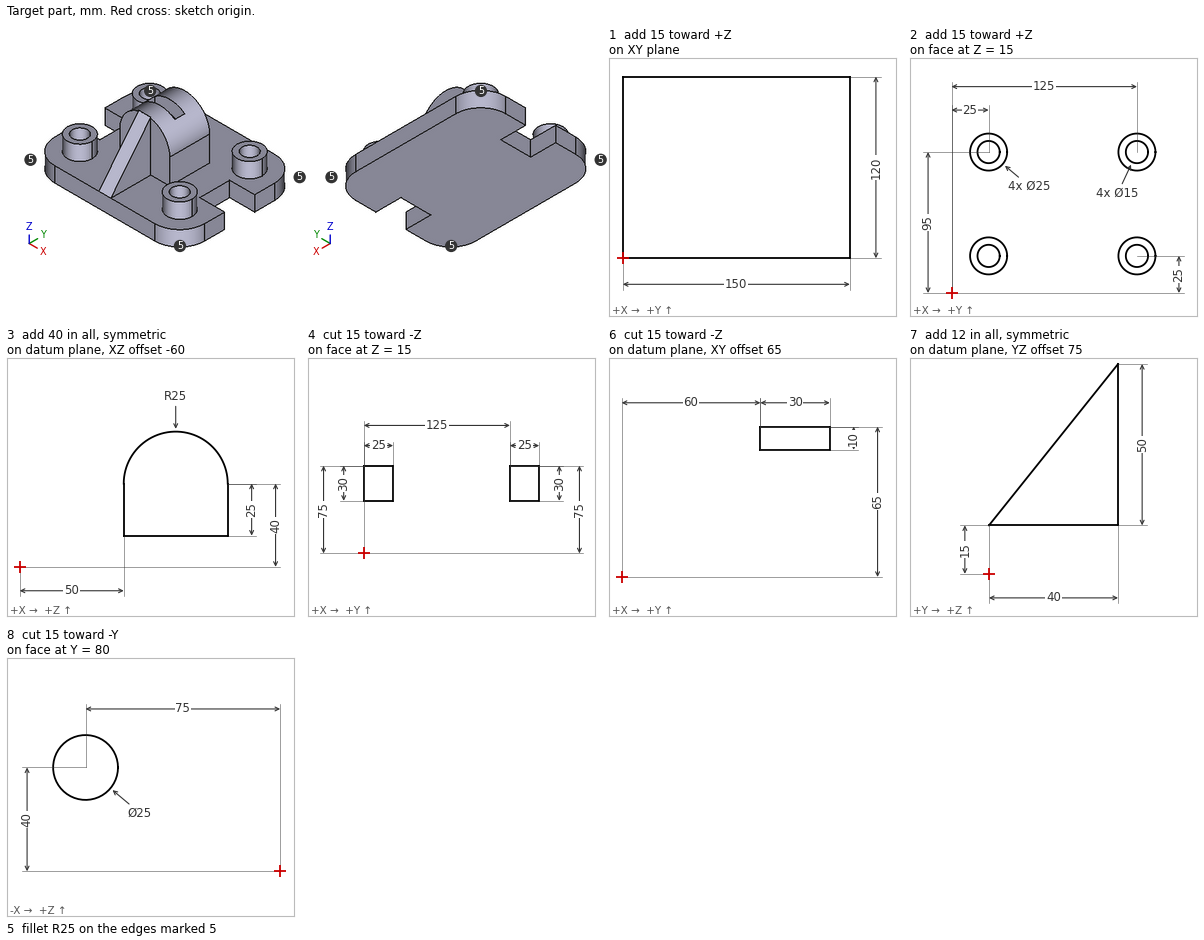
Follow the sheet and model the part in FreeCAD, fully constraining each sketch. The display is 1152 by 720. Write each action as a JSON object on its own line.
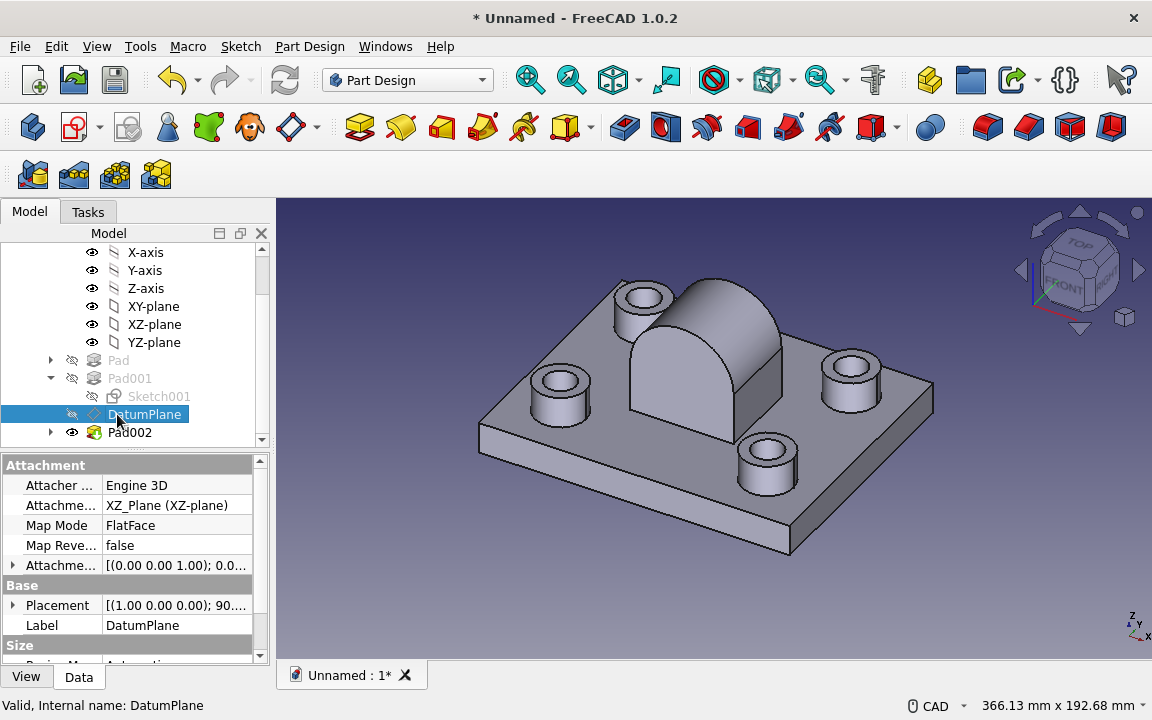
{"action": "left_click", "coordinate": [531, 80]}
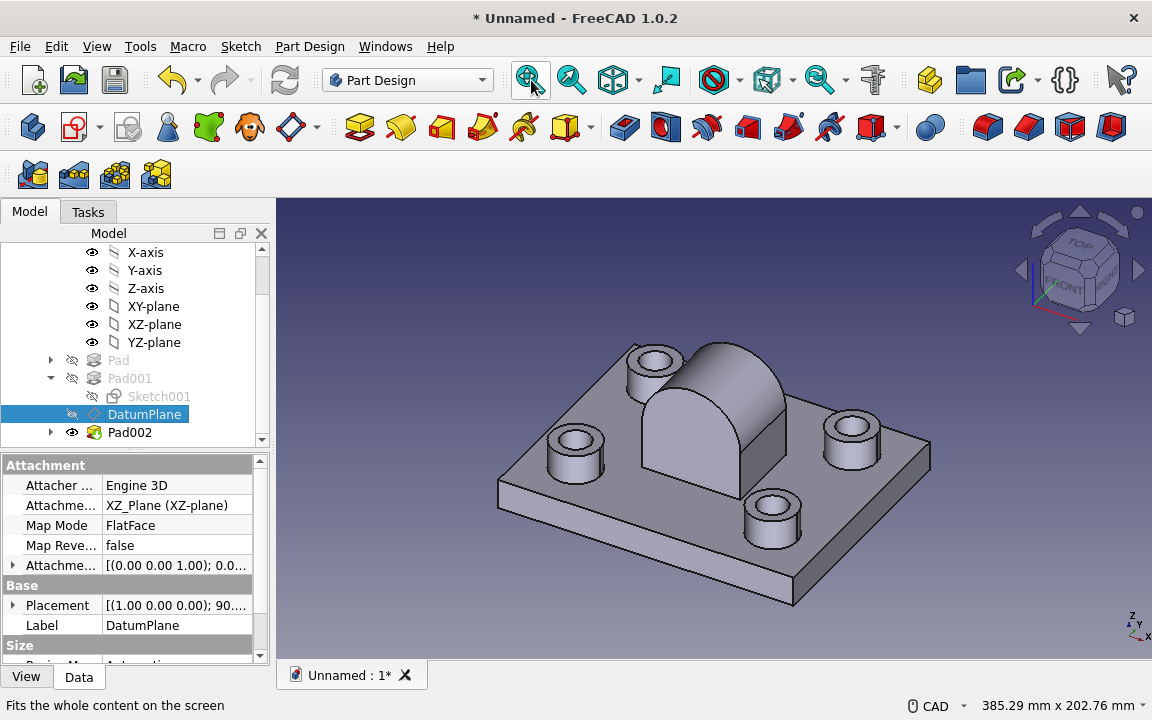
{"action": "left_click", "coordinate": [630, 432]}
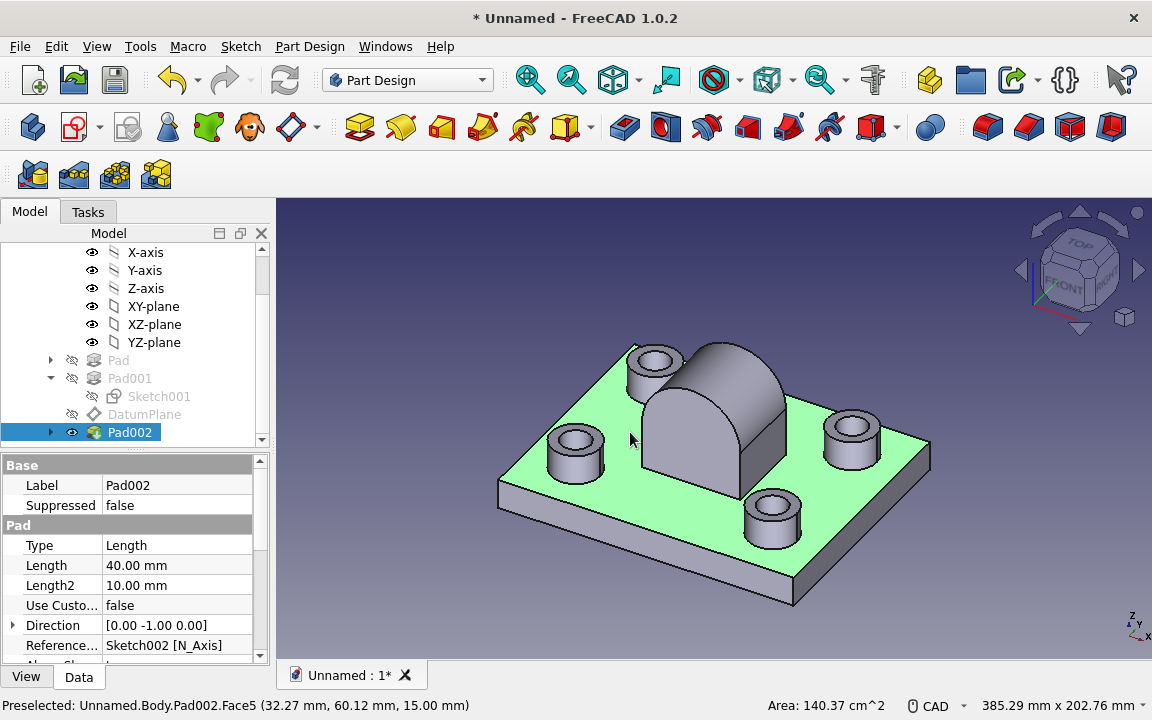
{"action": "left_click", "coordinate": [74, 128]}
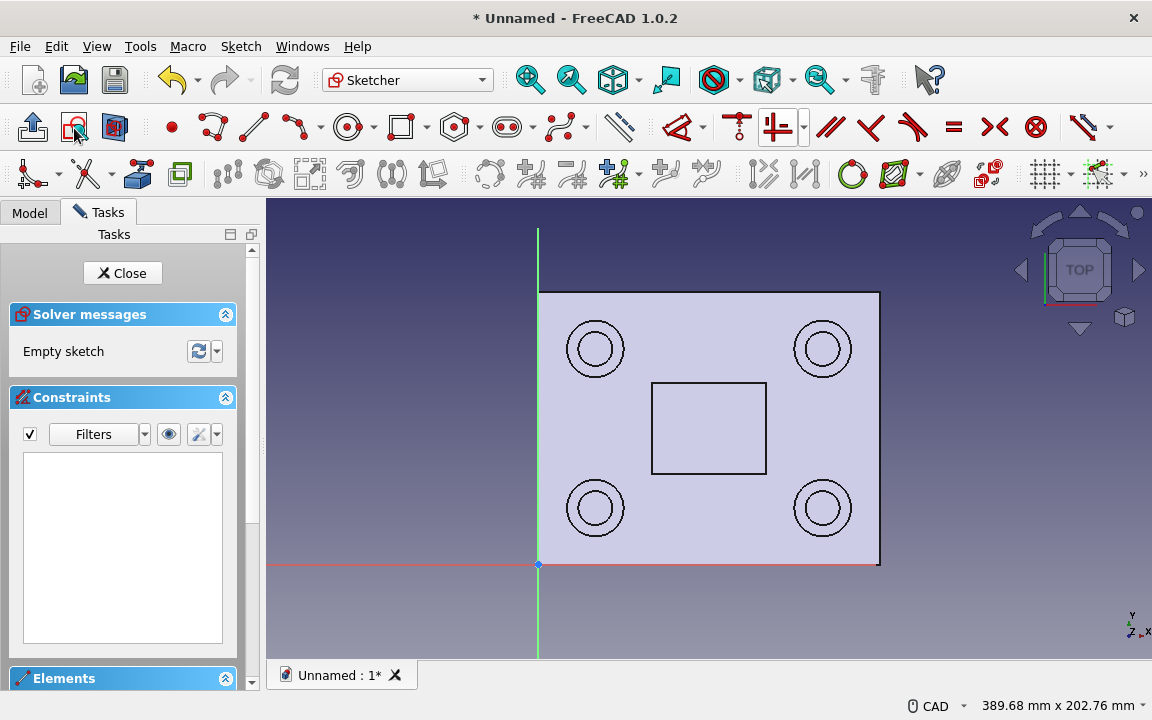
{"action": "left_click", "coordinate": [115, 128]}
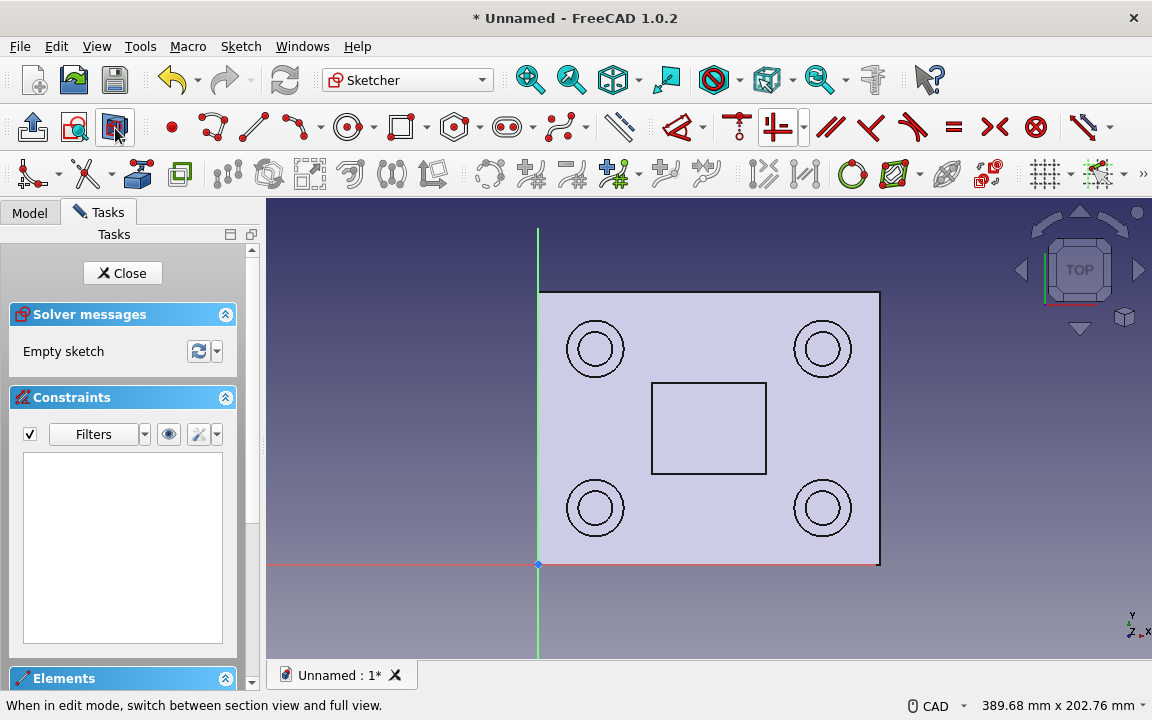
{"action": "scroll", "coordinate": [848, 584], "scroll_direction": "up", "scroll_amount": 2}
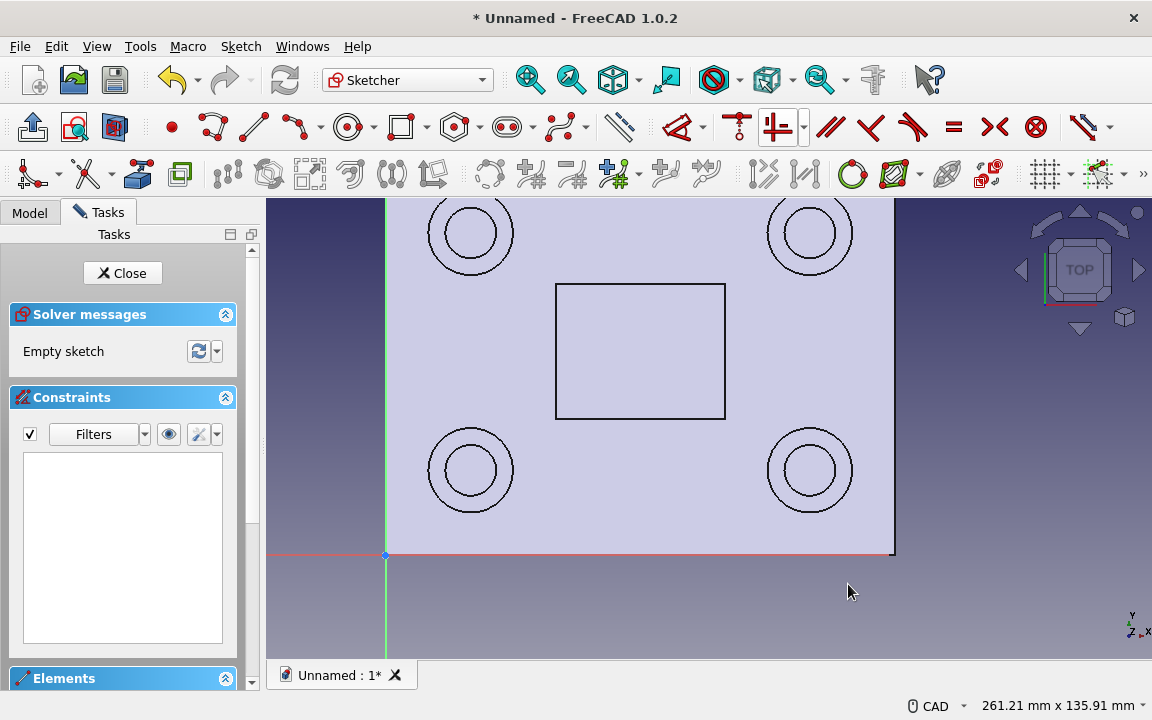
{"action": "left_click", "coordinate": [400, 128]}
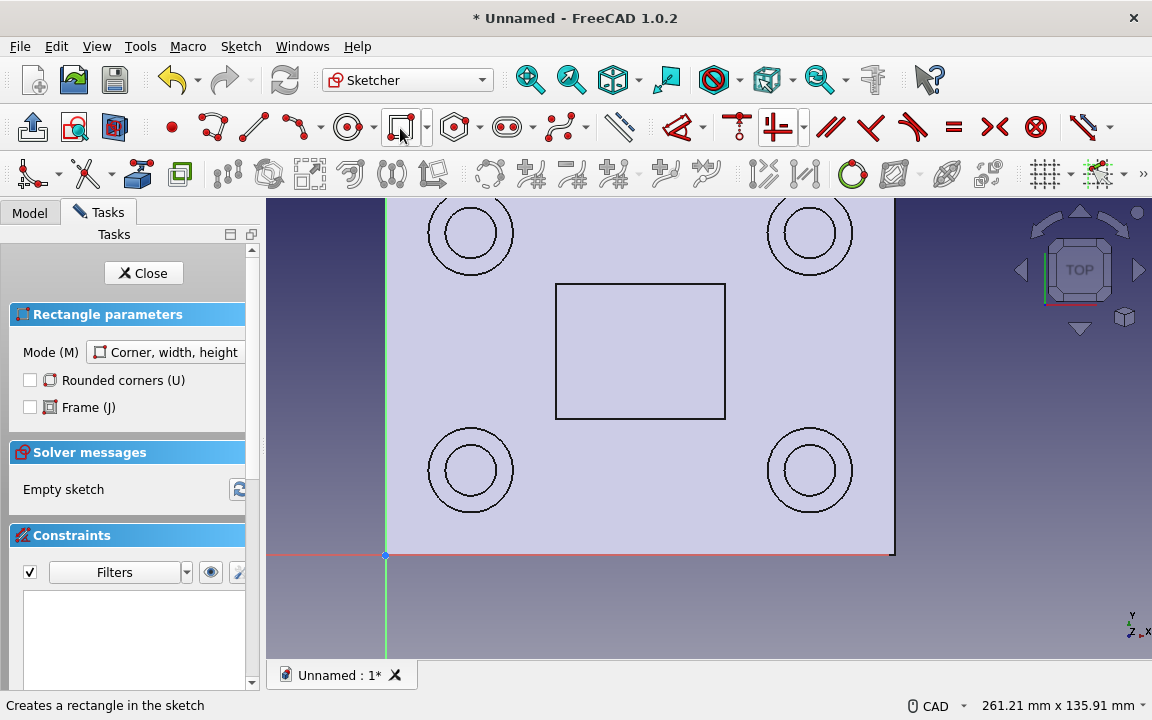
{"action": "left_click", "coordinate": [810, 301]}
{"action": "left_click", "coordinate": [895, 402]}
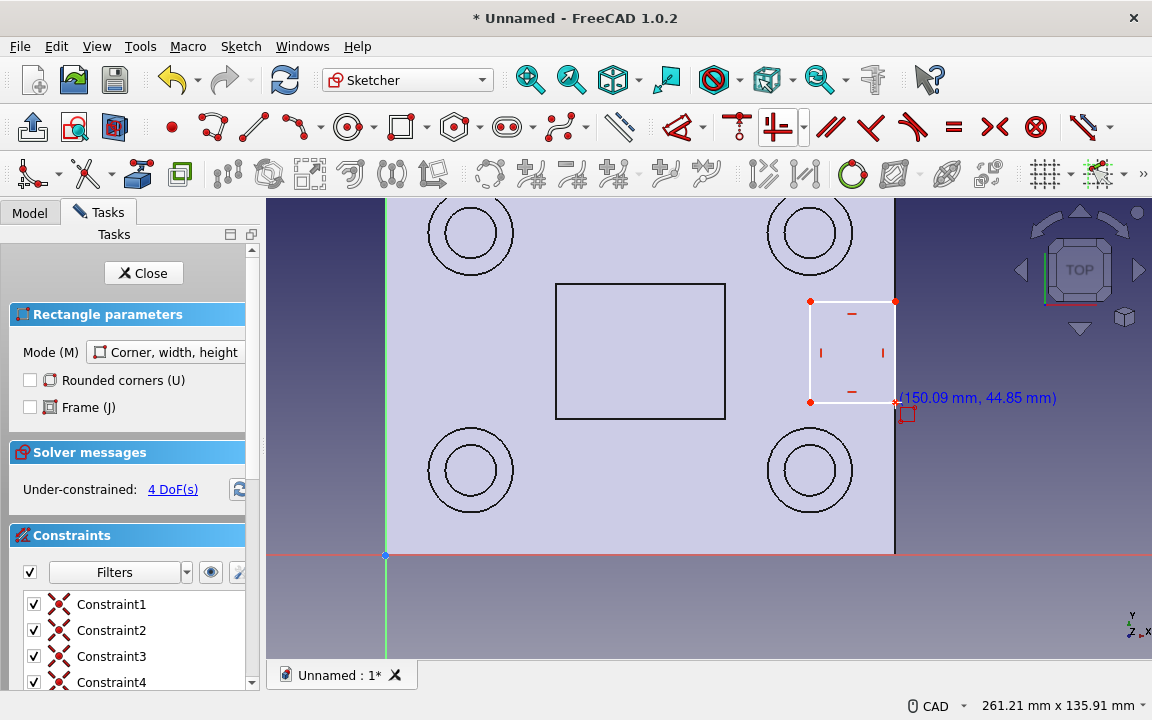
{"action": "left_click", "coordinate": [386, 301]}
{"action": "left_click", "coordinate": [471, 402]}
{"action": "key", "text": "Escape"}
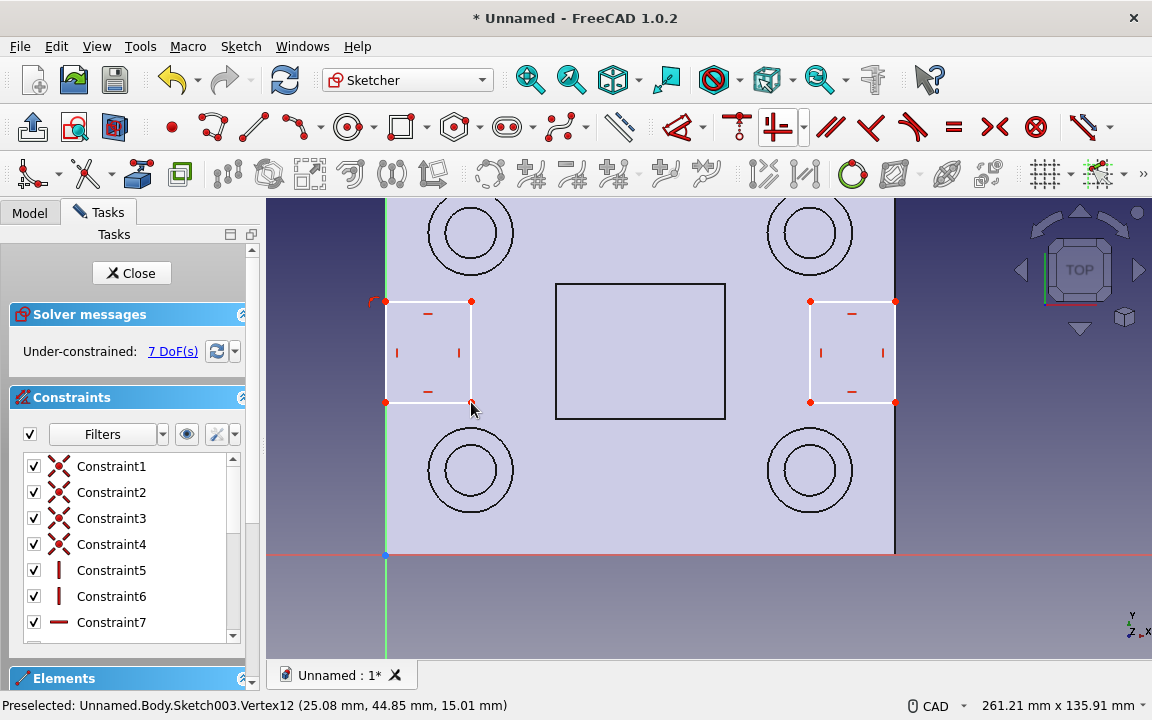
{"action": "left_click", "coordinate": [676, 128]}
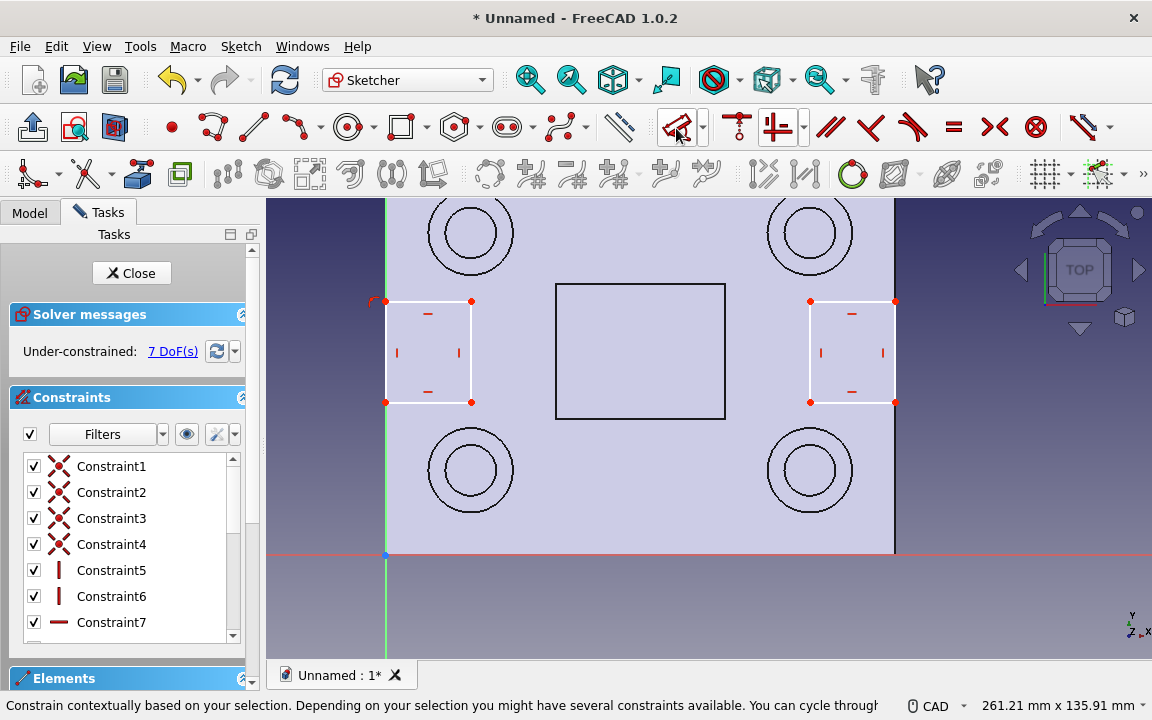
{"action": "left_click", "coordinate": [810, 332]}
{"action": "left_click", "coordinate": [844, 352]}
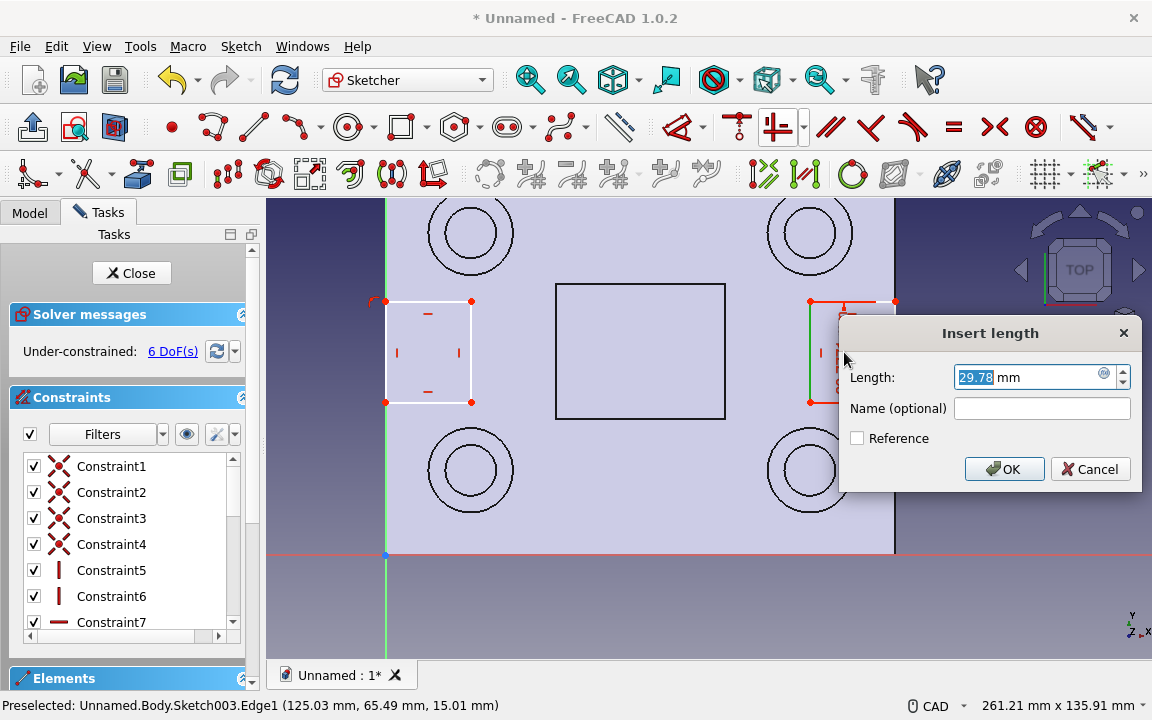
{"action": "type", "text": "30"}
{"action": "key", "text": "Return"}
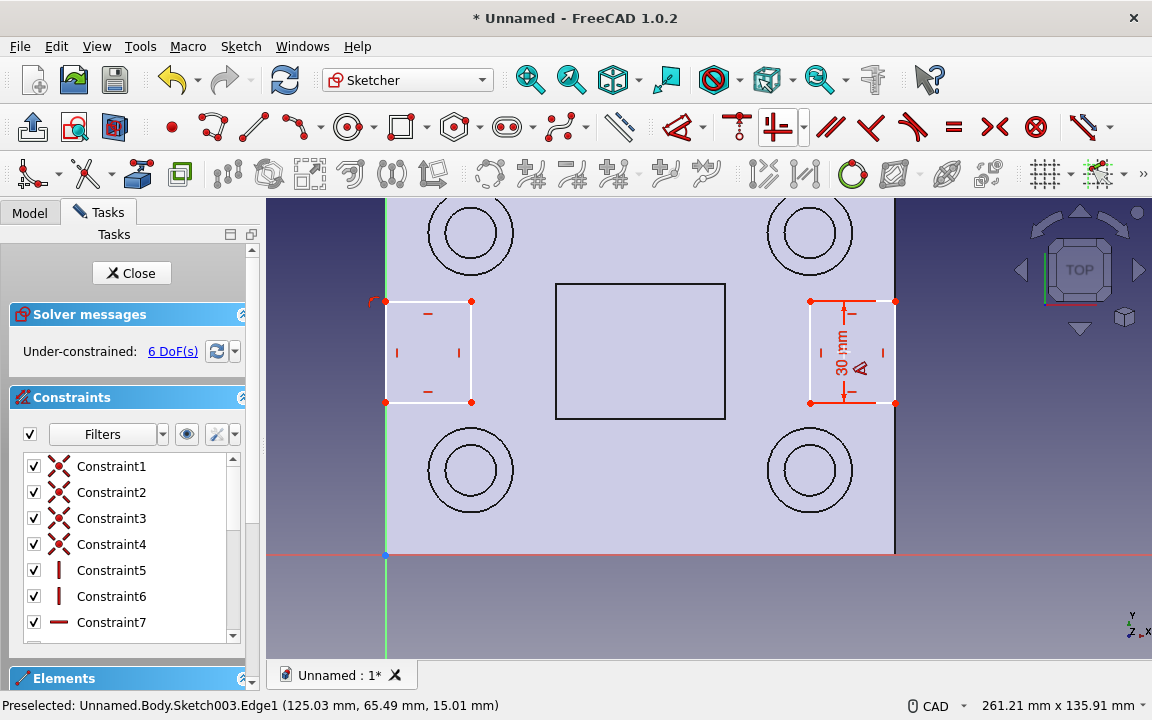
{"action": "left_click", "coordinate": [836, 403]}
{"action": "left_click", "coordinate": [853, 437]}